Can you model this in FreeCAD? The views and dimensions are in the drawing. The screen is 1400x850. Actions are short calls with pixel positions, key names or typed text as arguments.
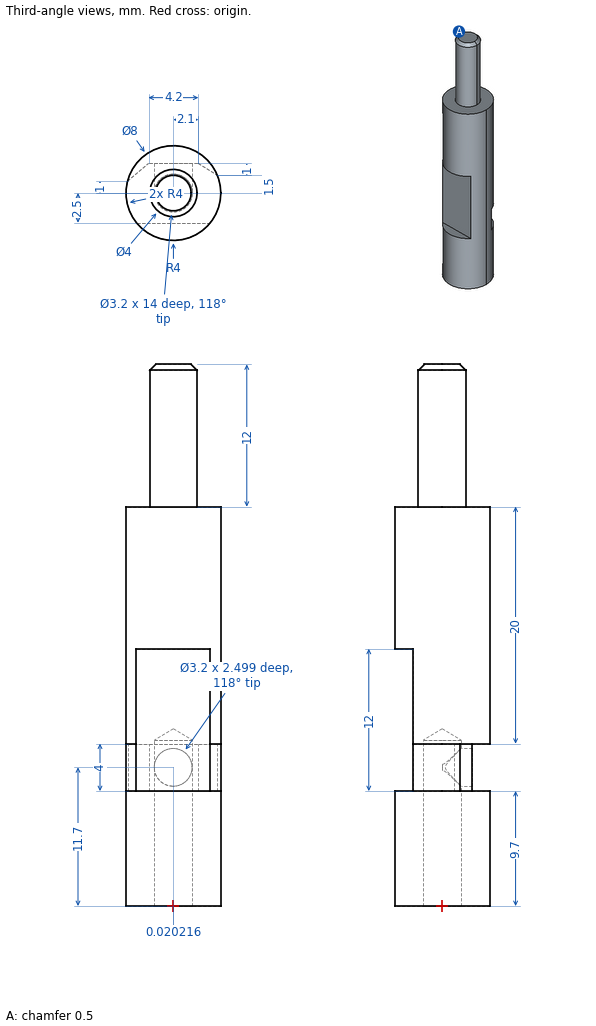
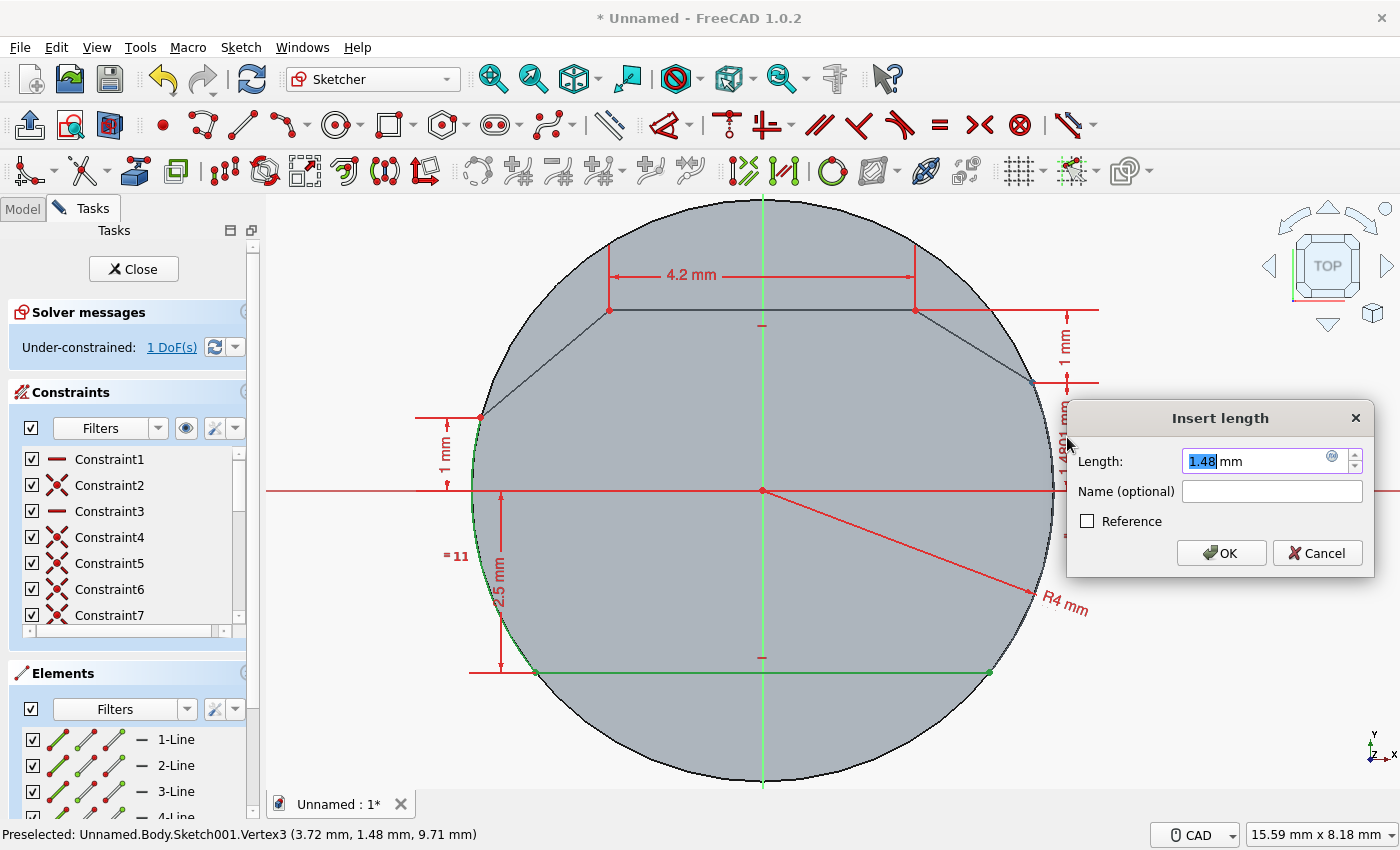
text(1.5)
key(Return)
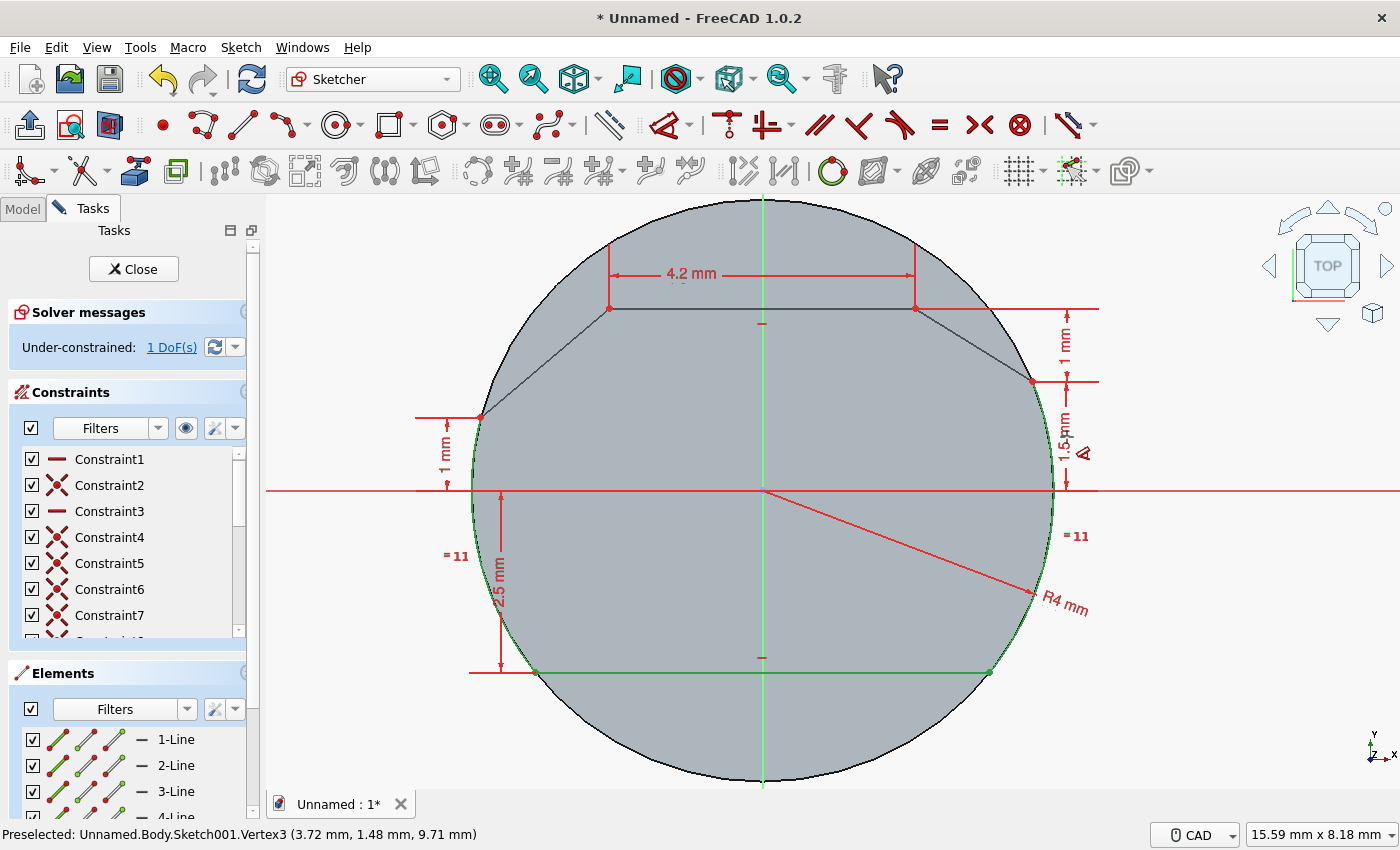
click(915, 309)
click(839, 275)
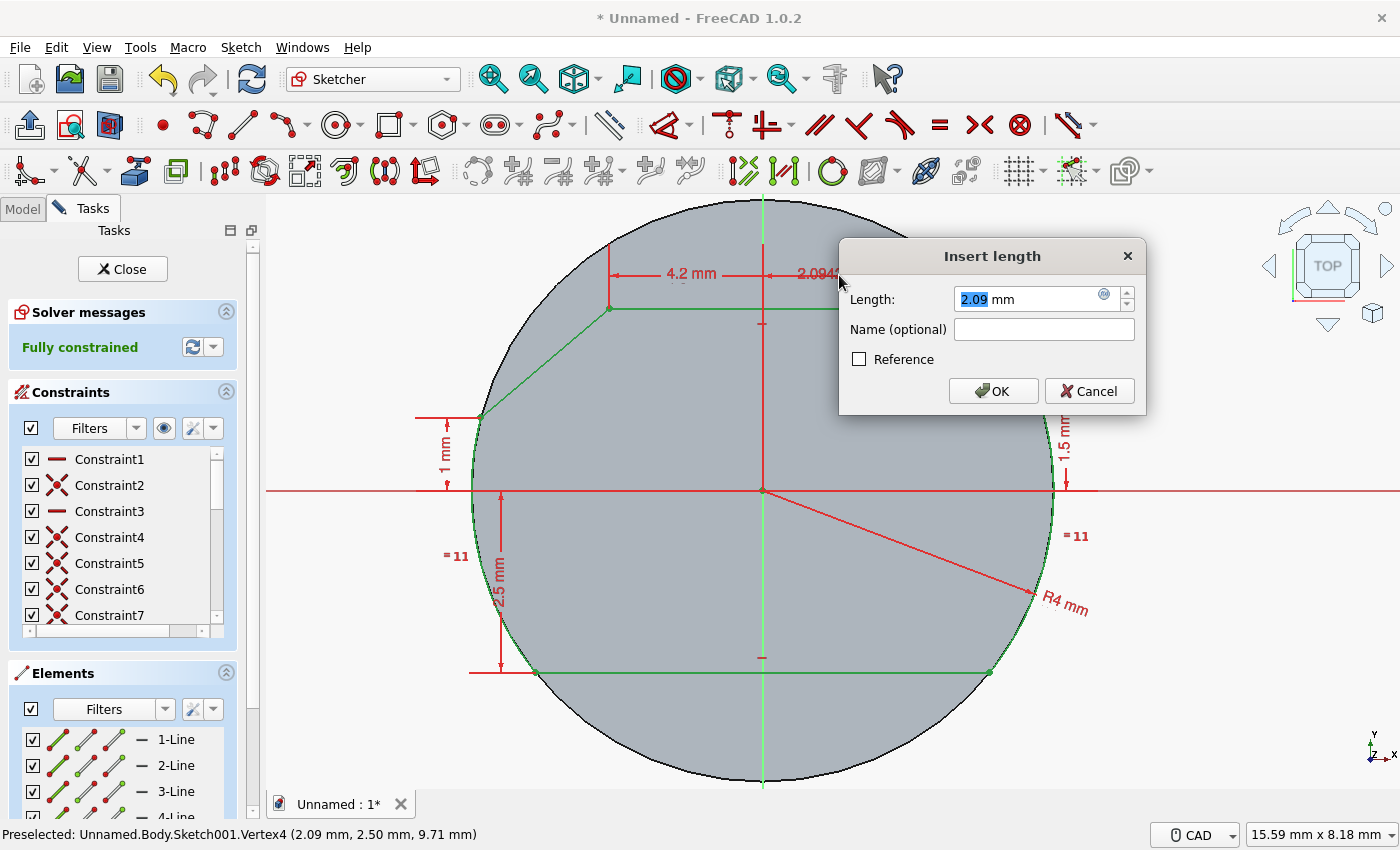
text(2.1)
key(Return)
key(Escape)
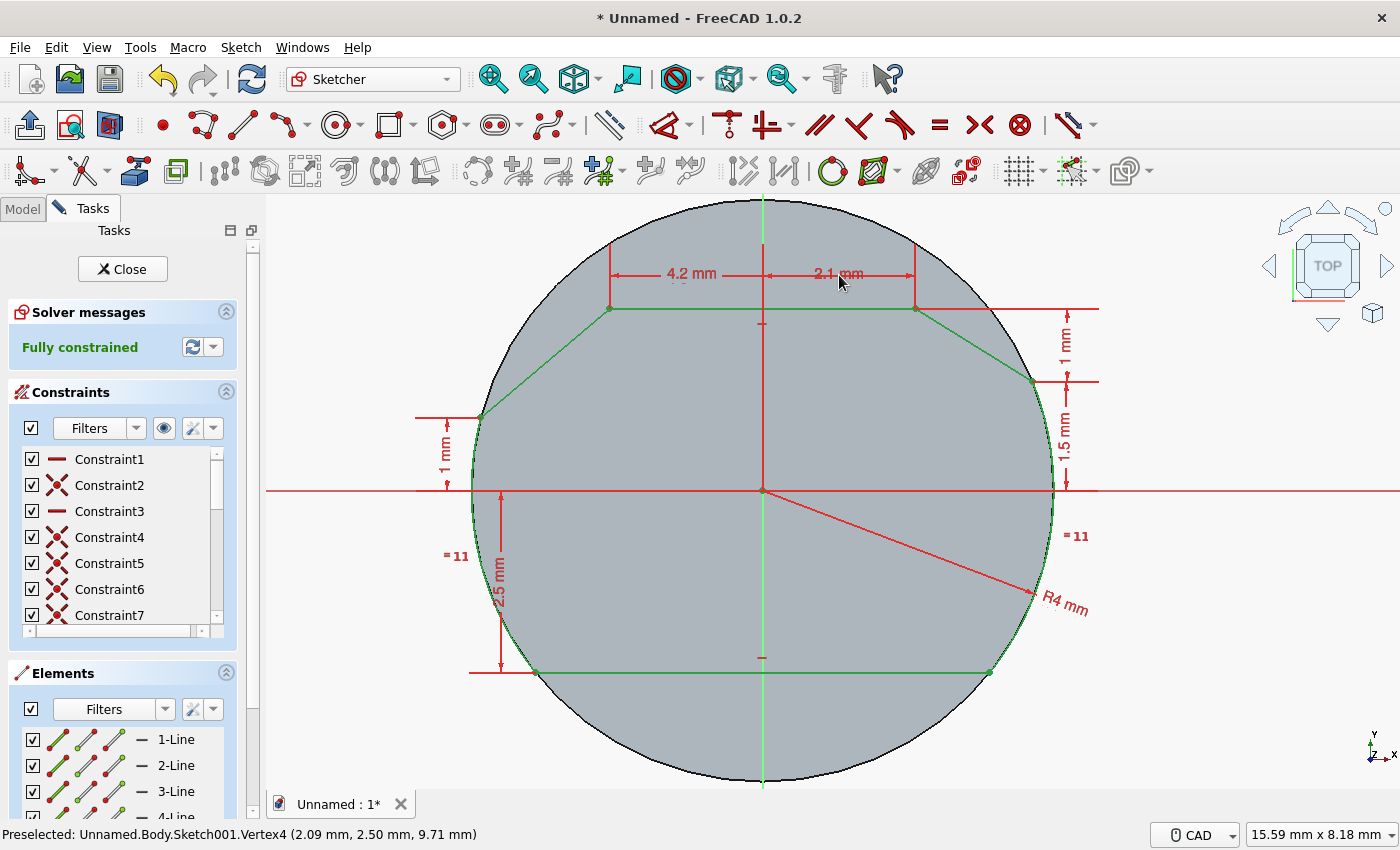
click(123, 269)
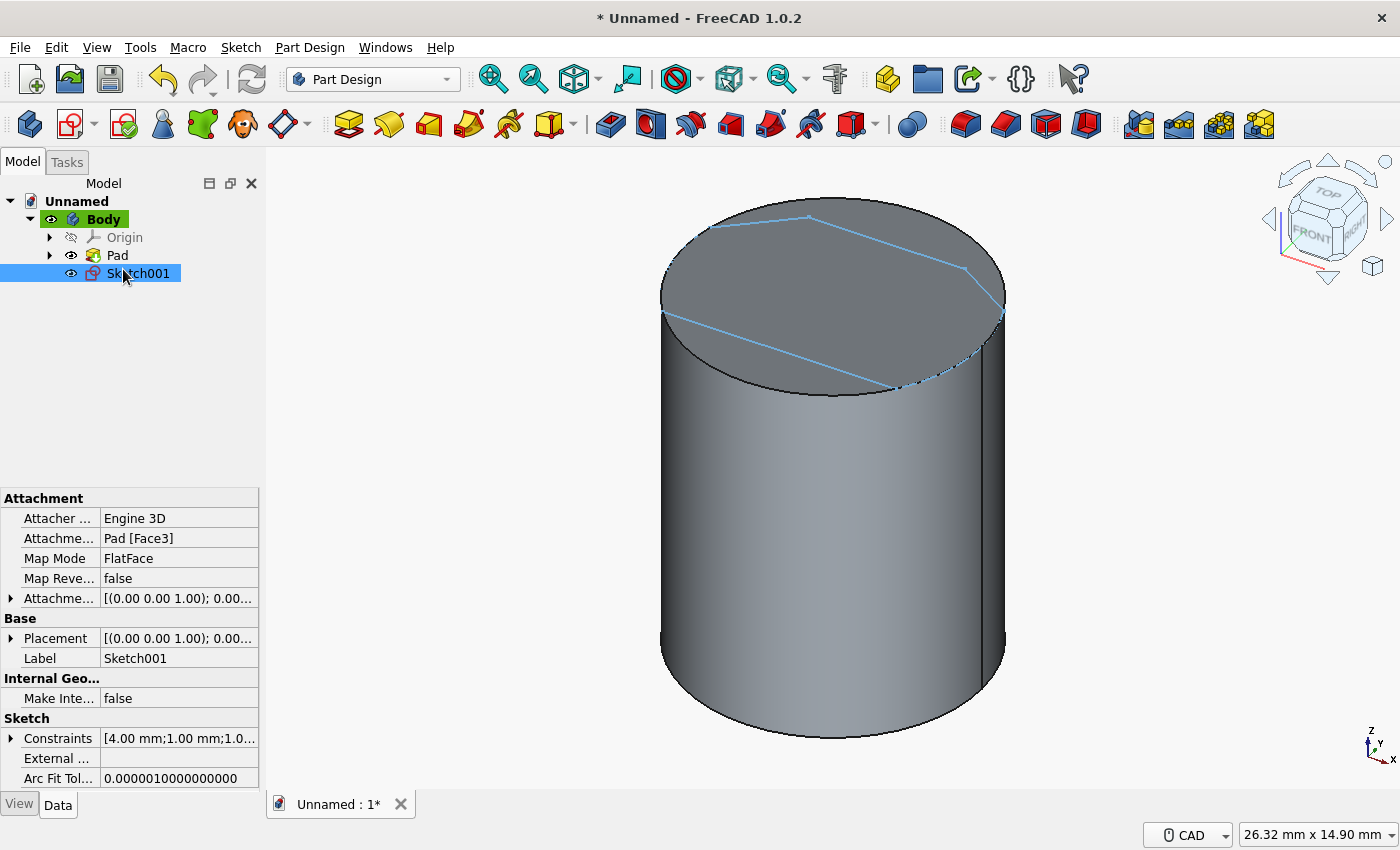
click(350, 124)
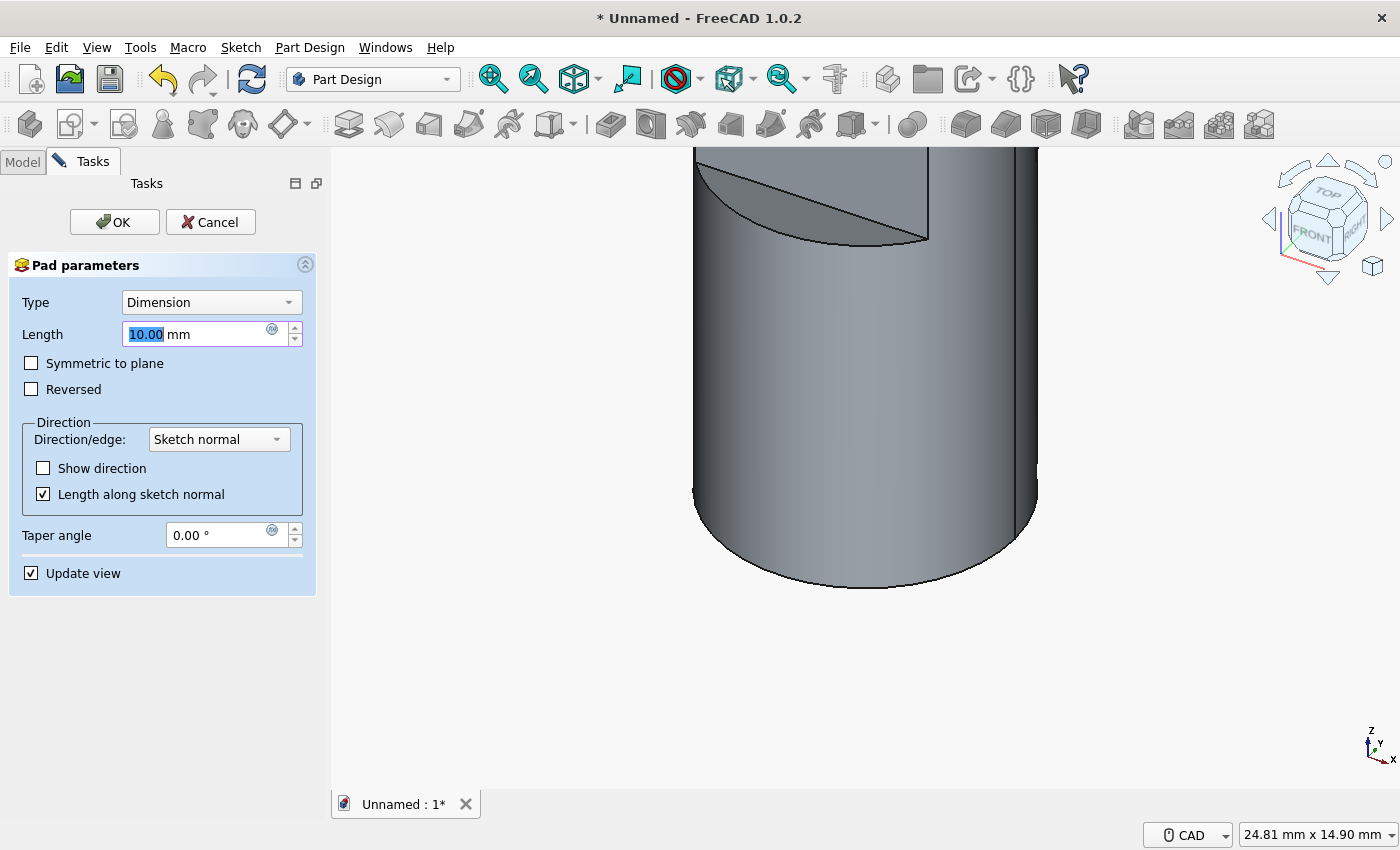
text(4)
key(Tab)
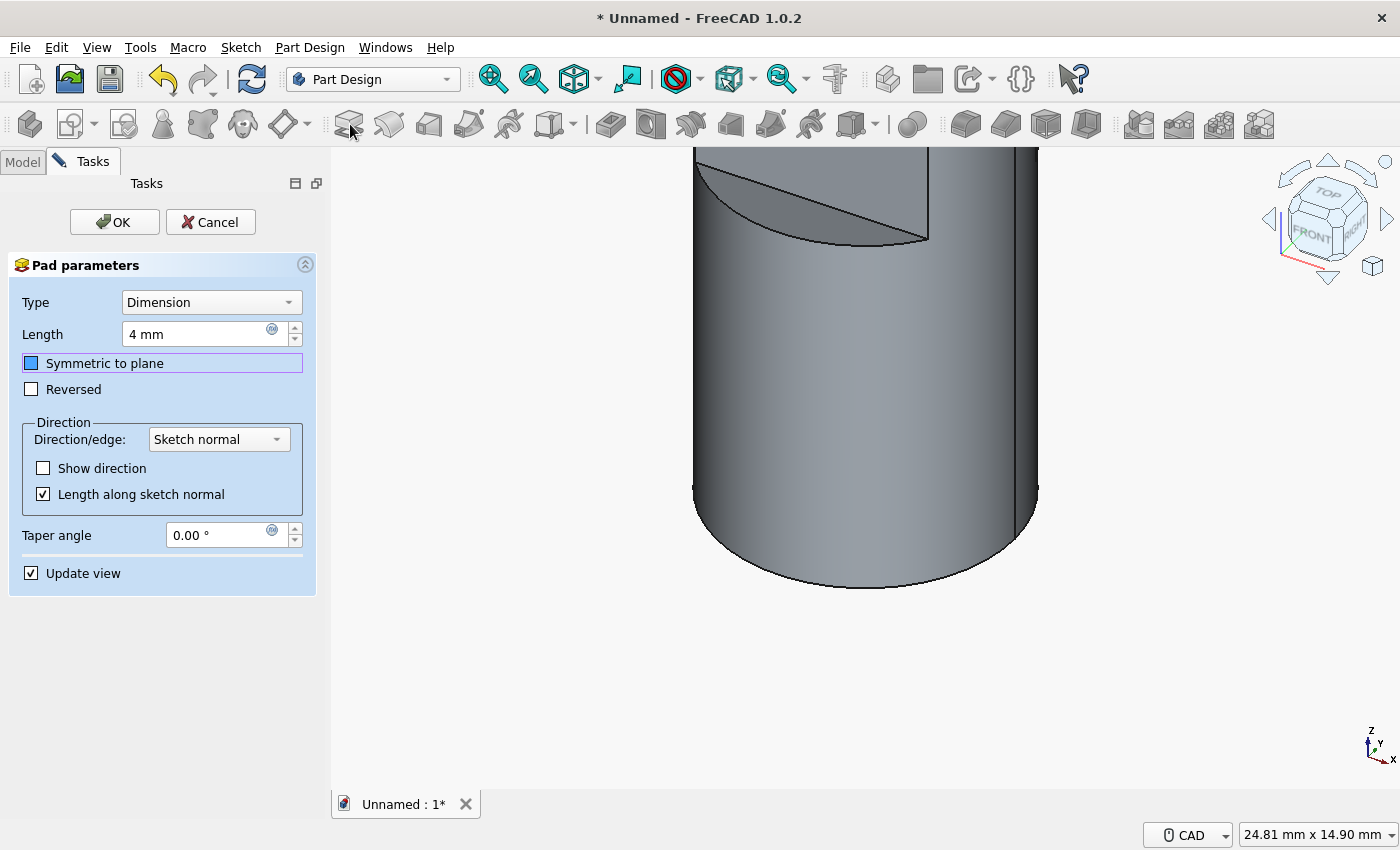
click(115, 222)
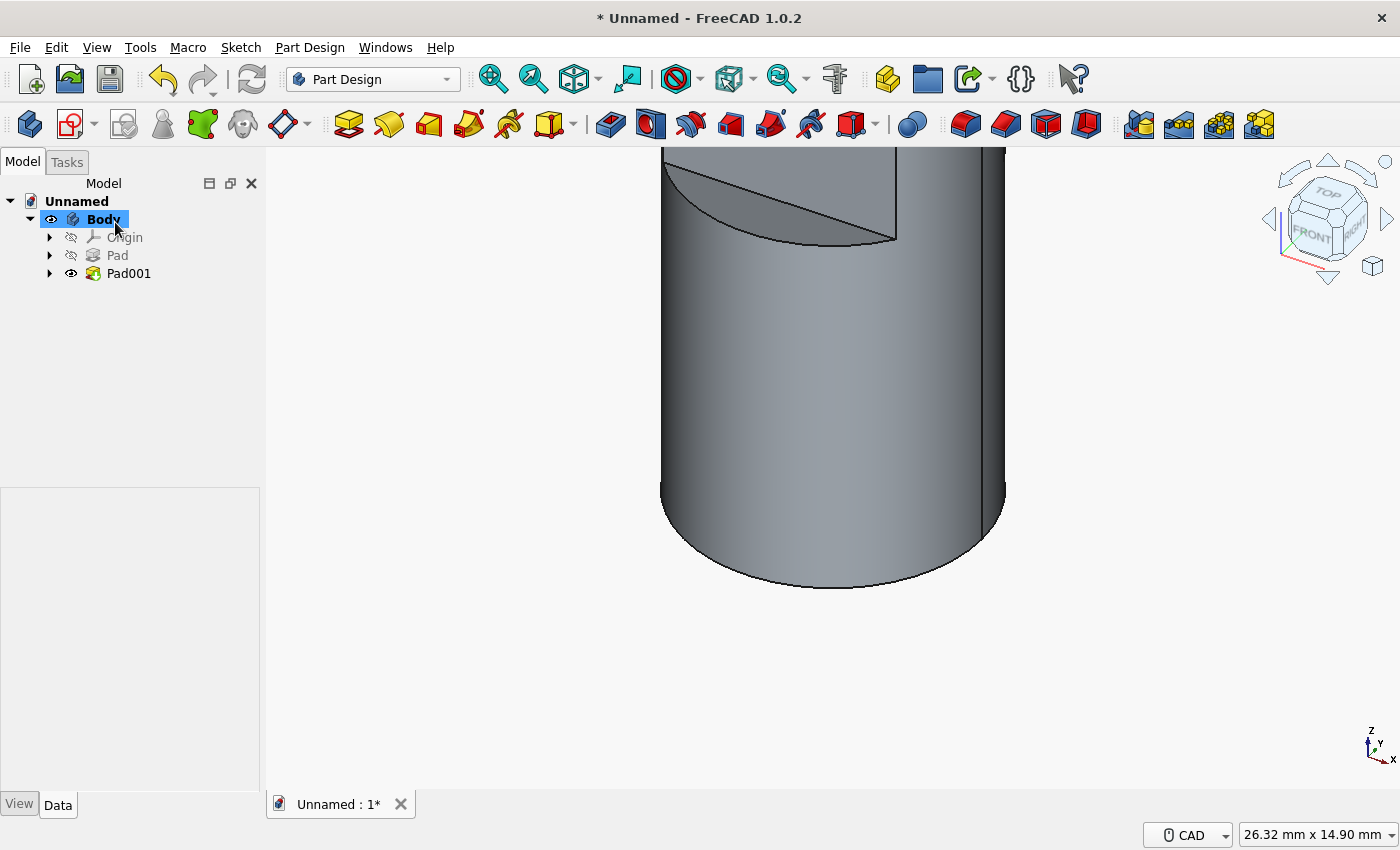
key(v)
key(f)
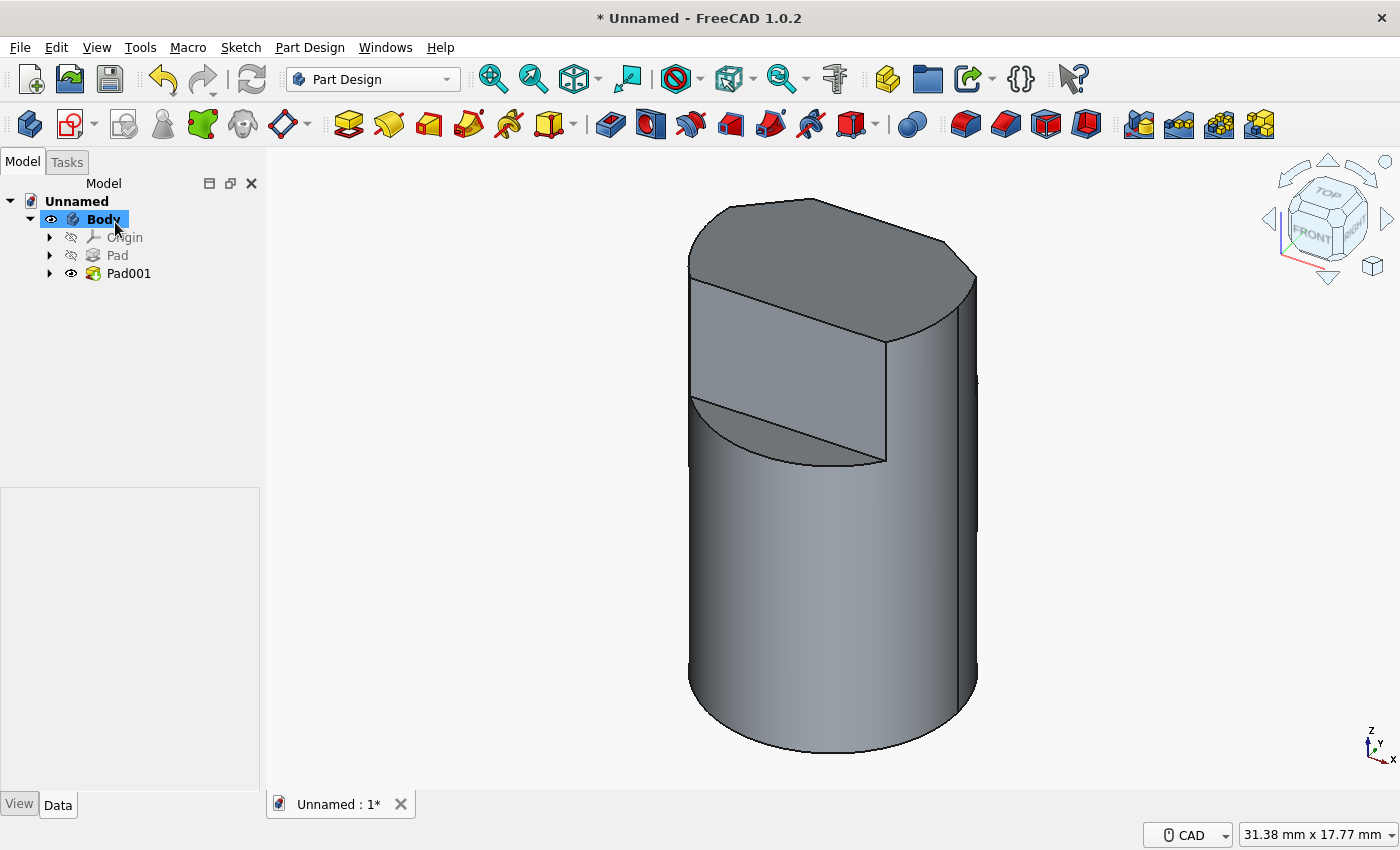
click(869, 276)